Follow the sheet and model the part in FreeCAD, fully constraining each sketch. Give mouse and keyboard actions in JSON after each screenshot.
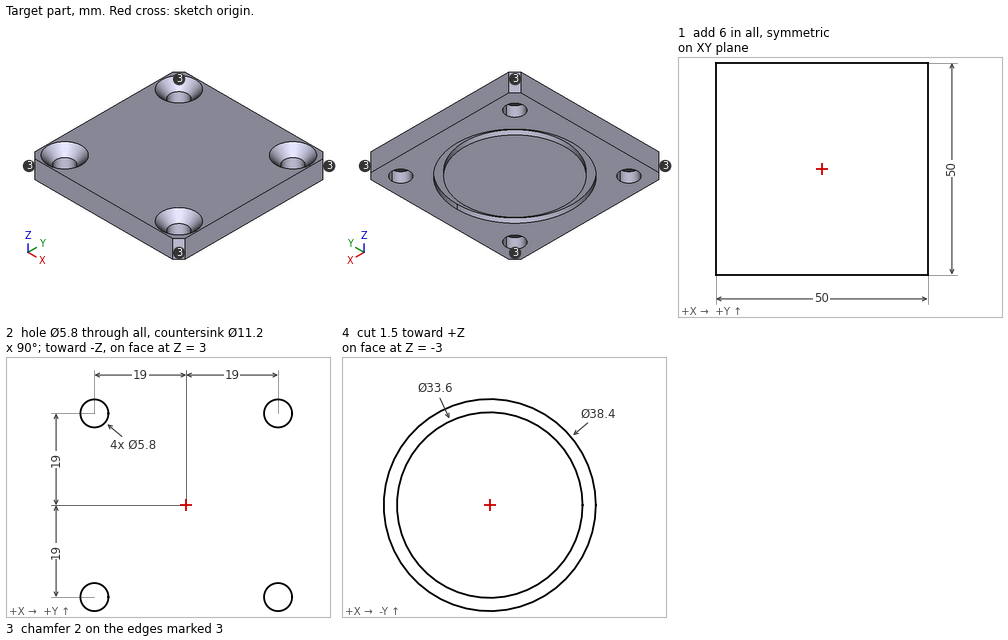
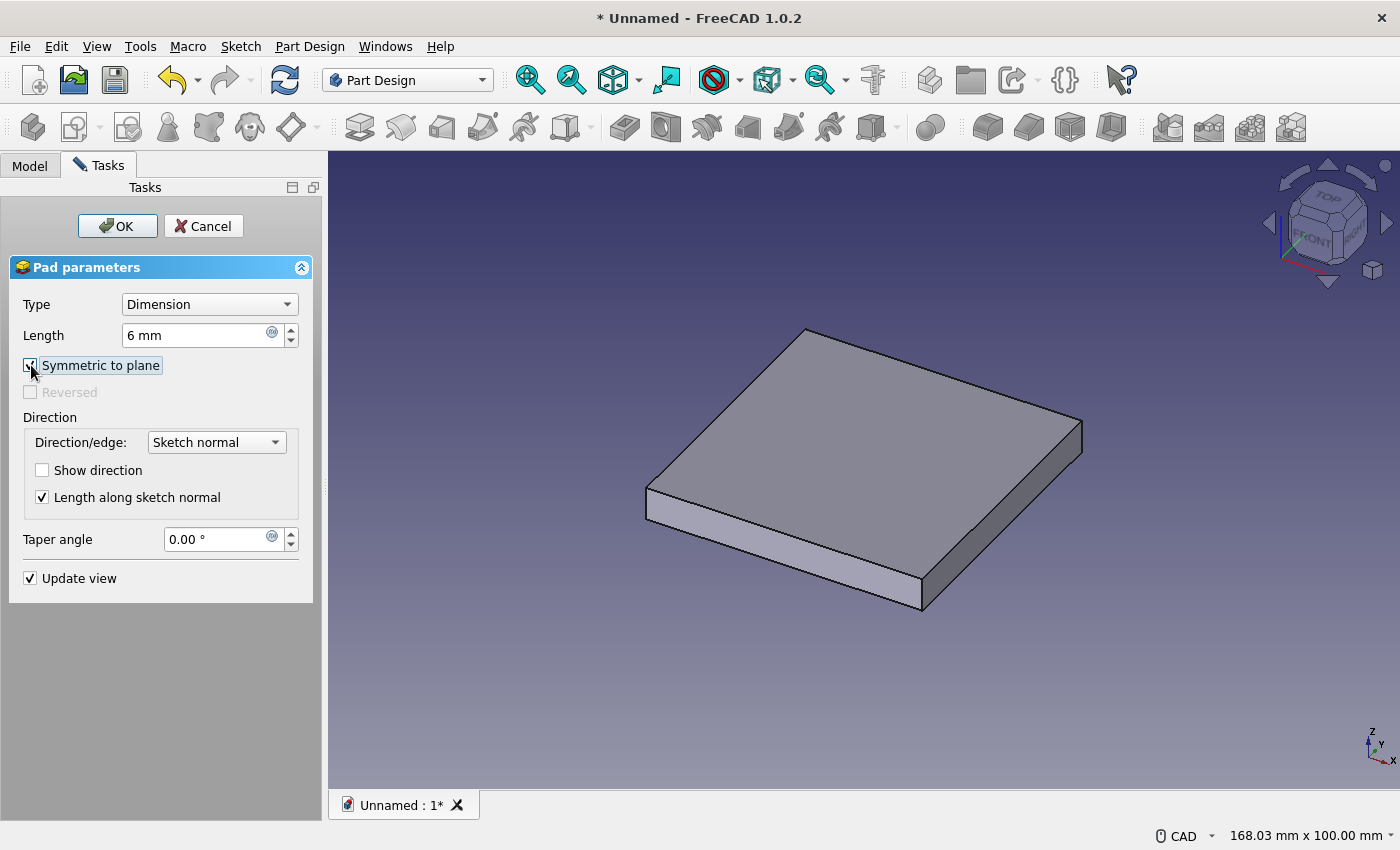
{"action": "left_click", "coordinate": [118, 226]}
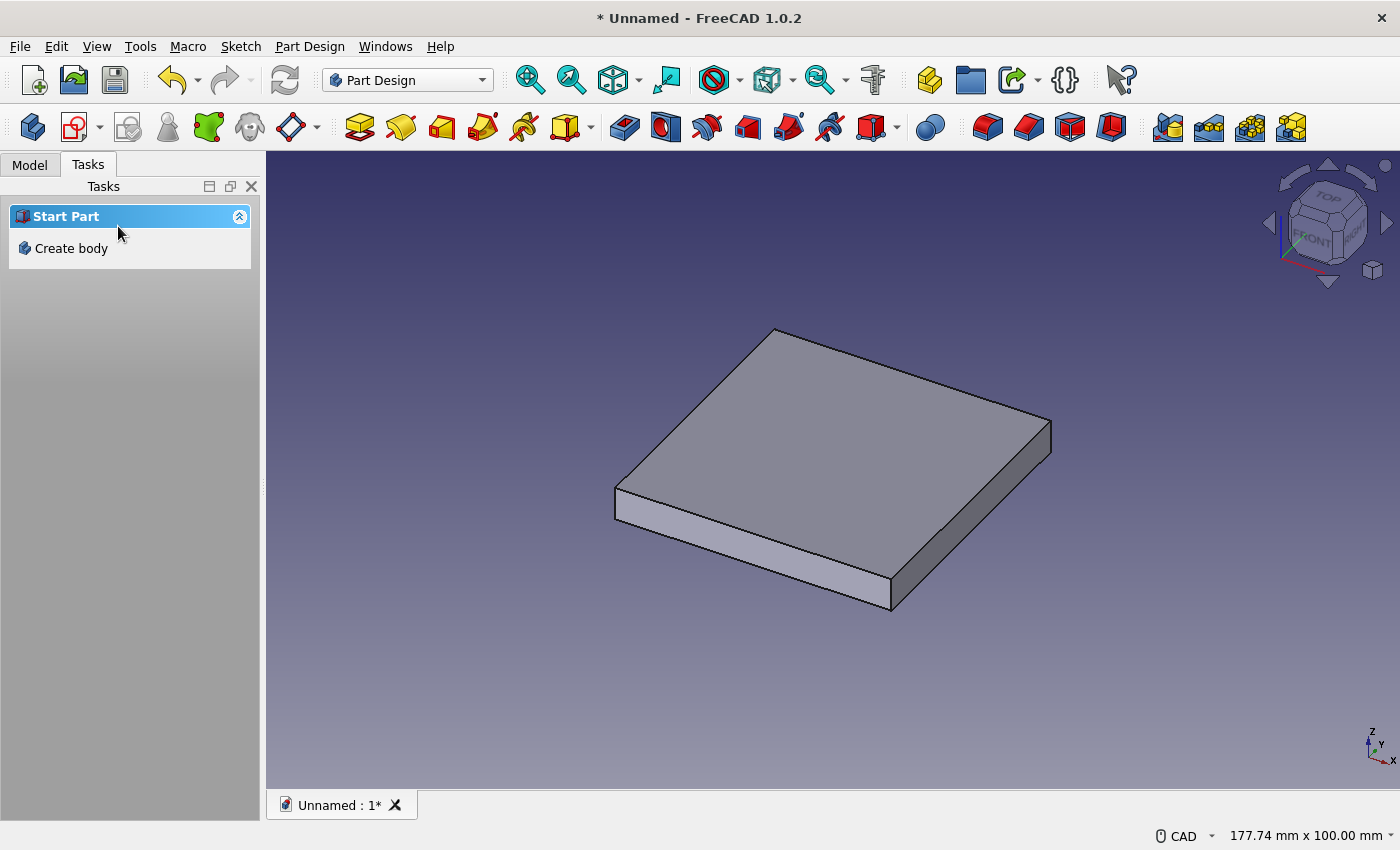
{"action": "left_click", "coordinate": [531, 80]}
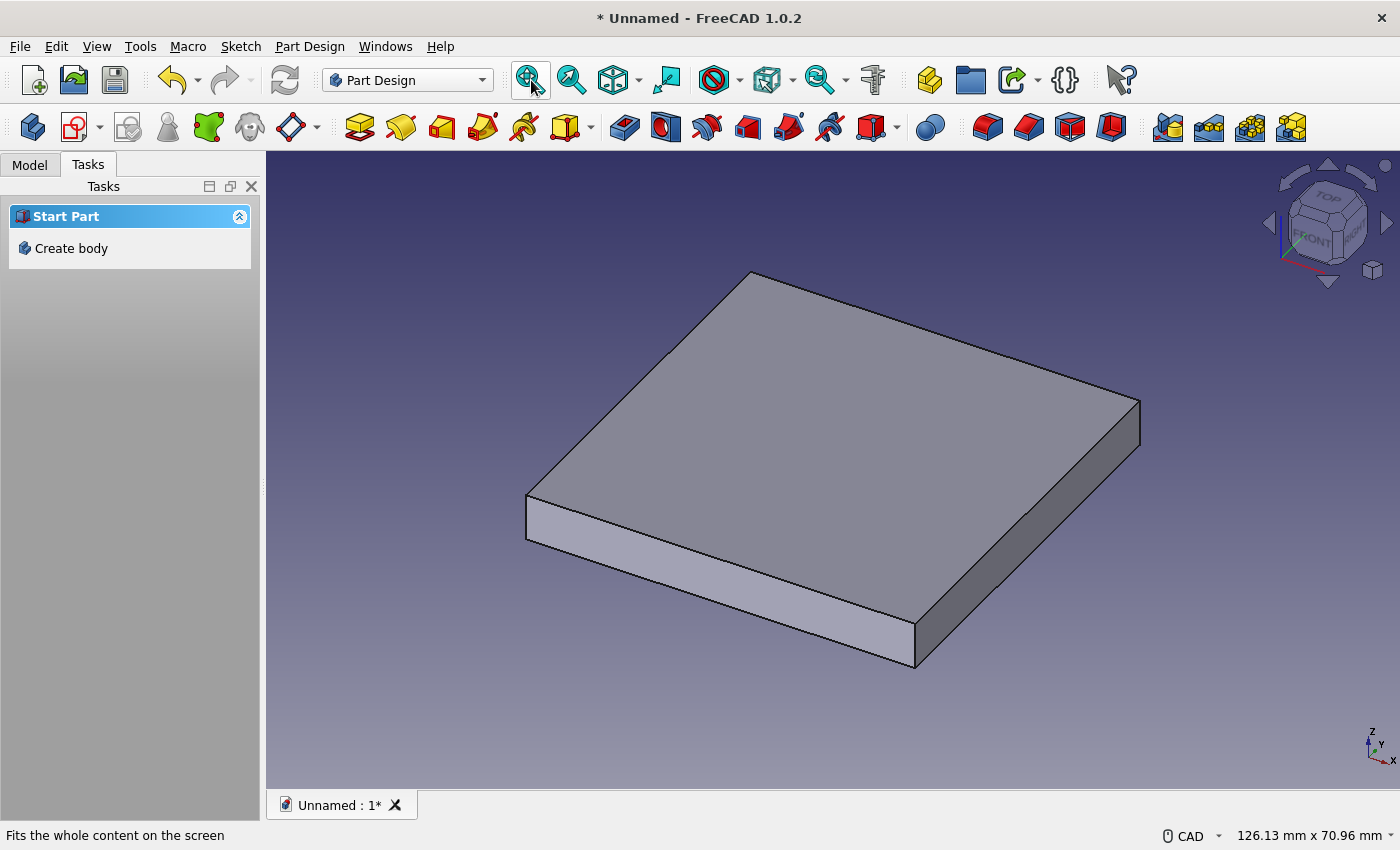
{"action": "left_click", "coordinate": [833, 447]}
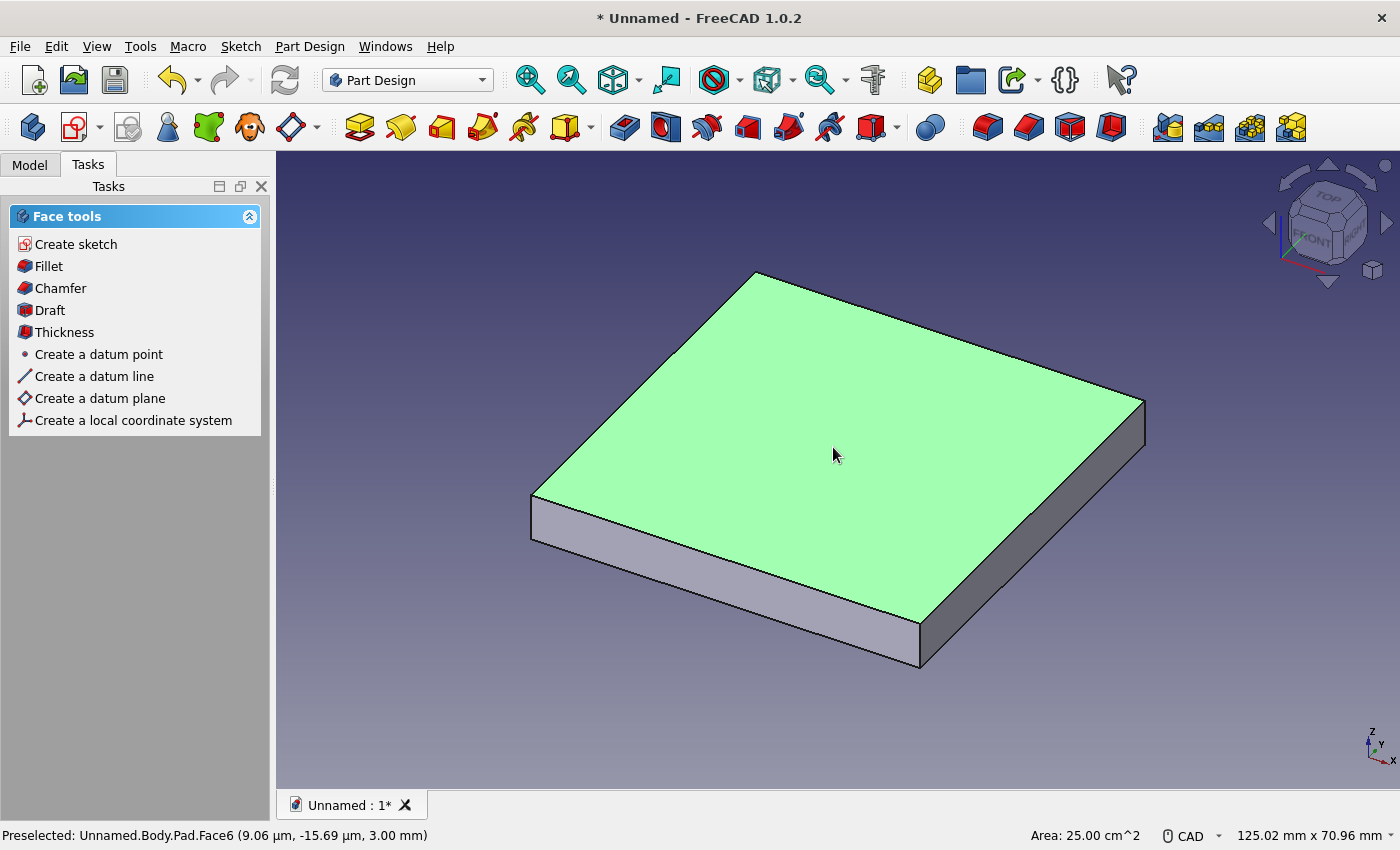
{"action": "left_click", "coordinate": [74, 128]}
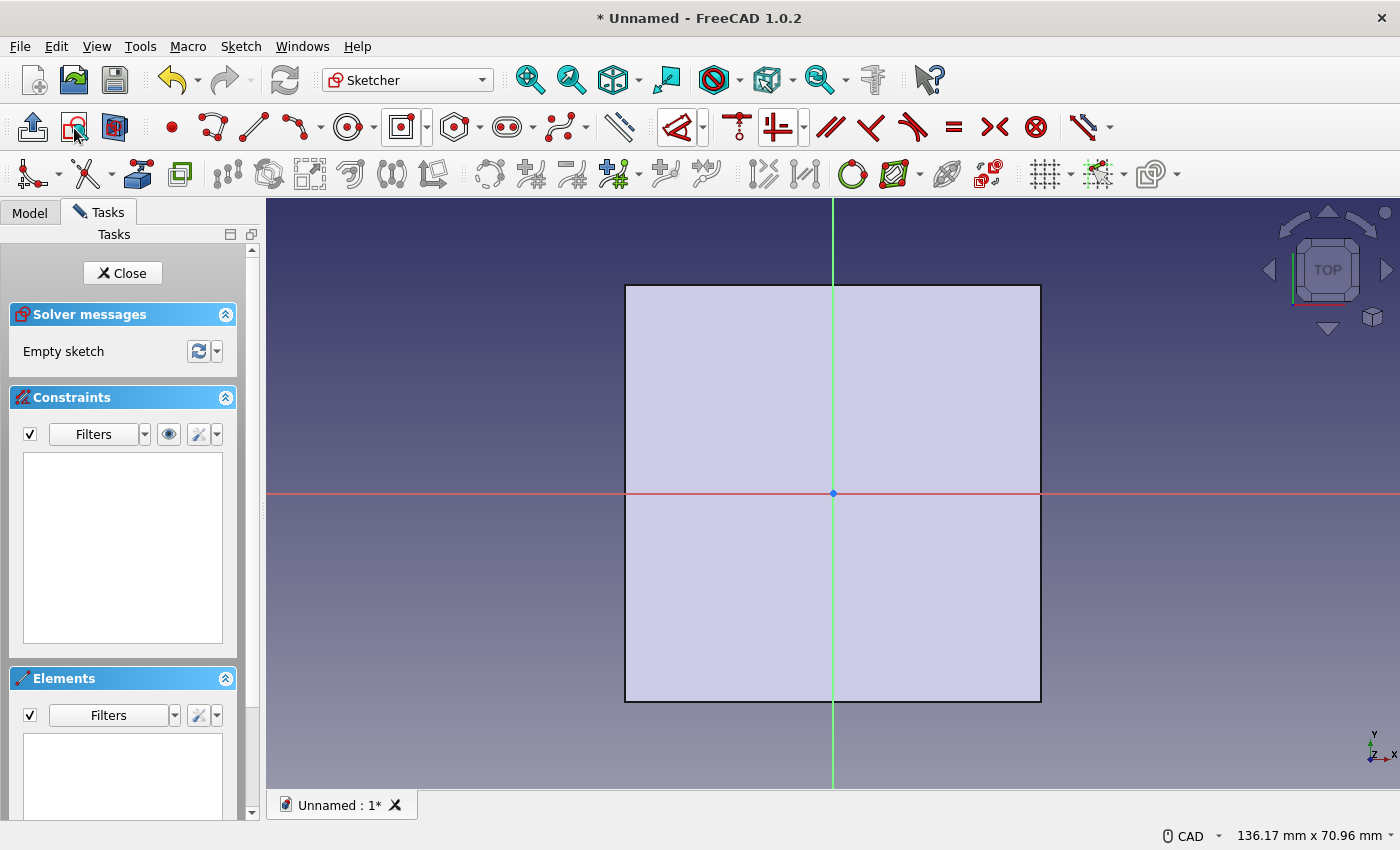
{"action": "left_click", "coordinate": [348, 128]}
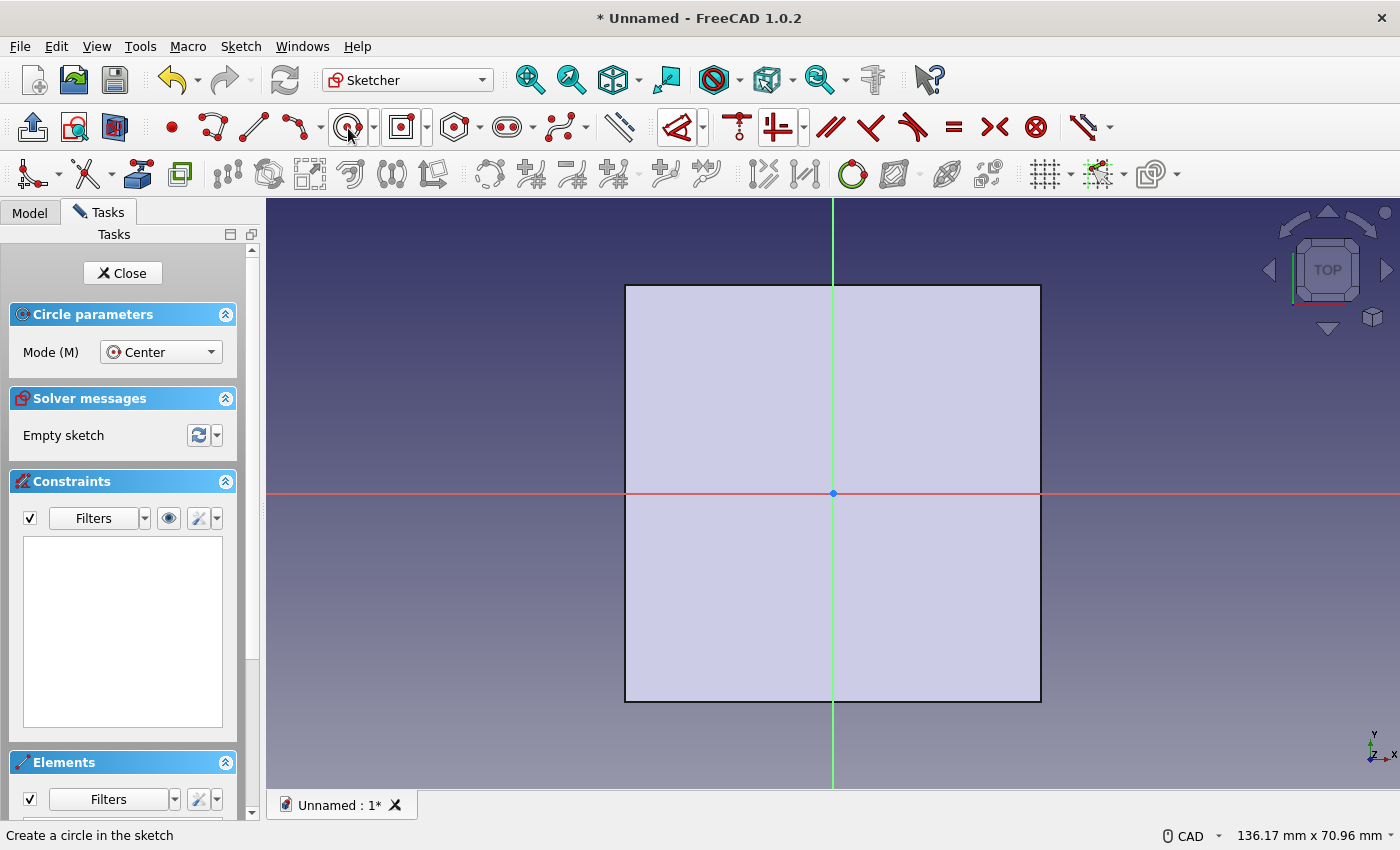
{"action": "left_click", "coordinate": [675, 335]}
{"action": "left_click", "coordinate": [692, 318]}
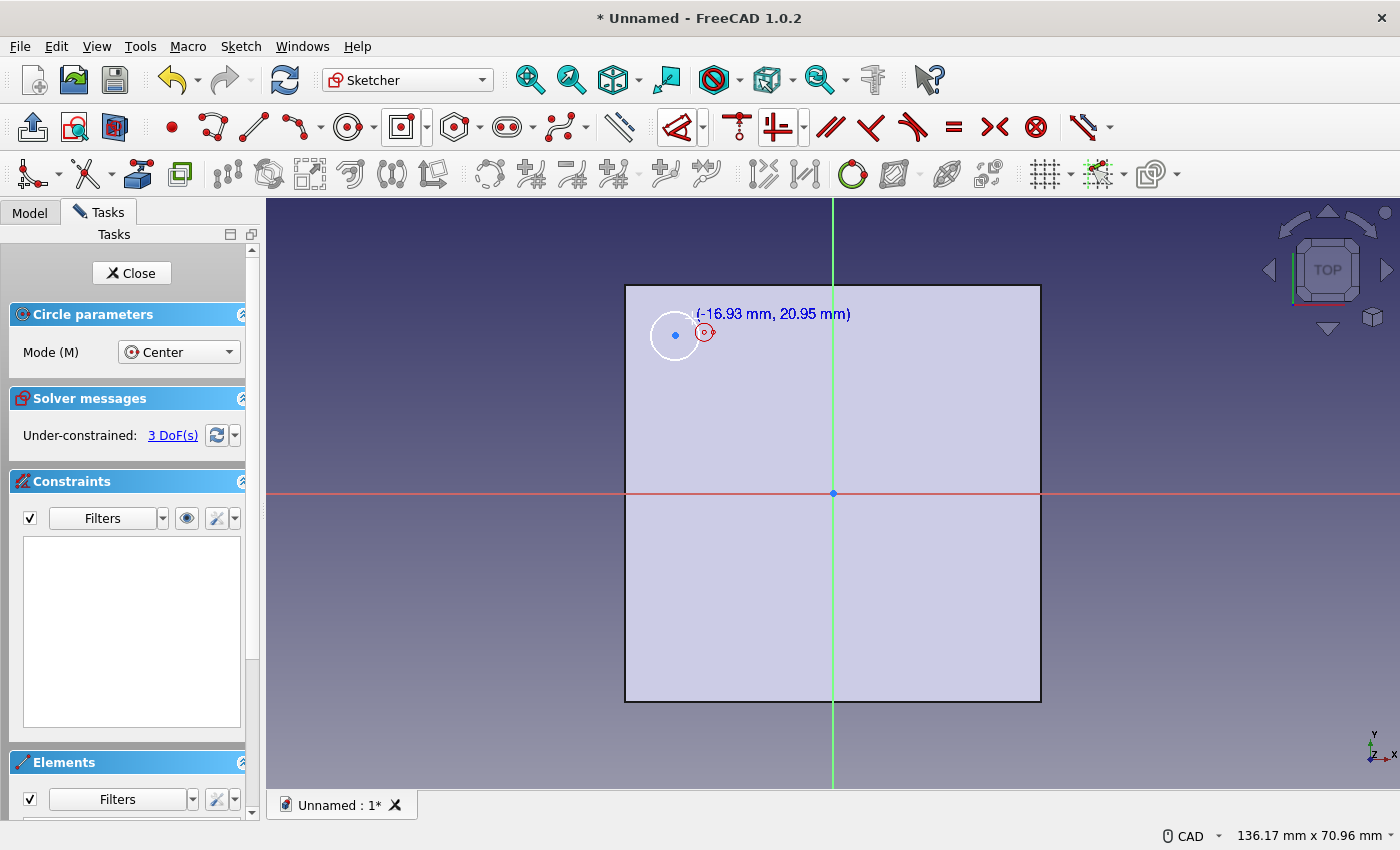
{"action": "left_click", "coordinate": [991, 335]}
{"action": "left_click", "coordinate": [1008, 318]}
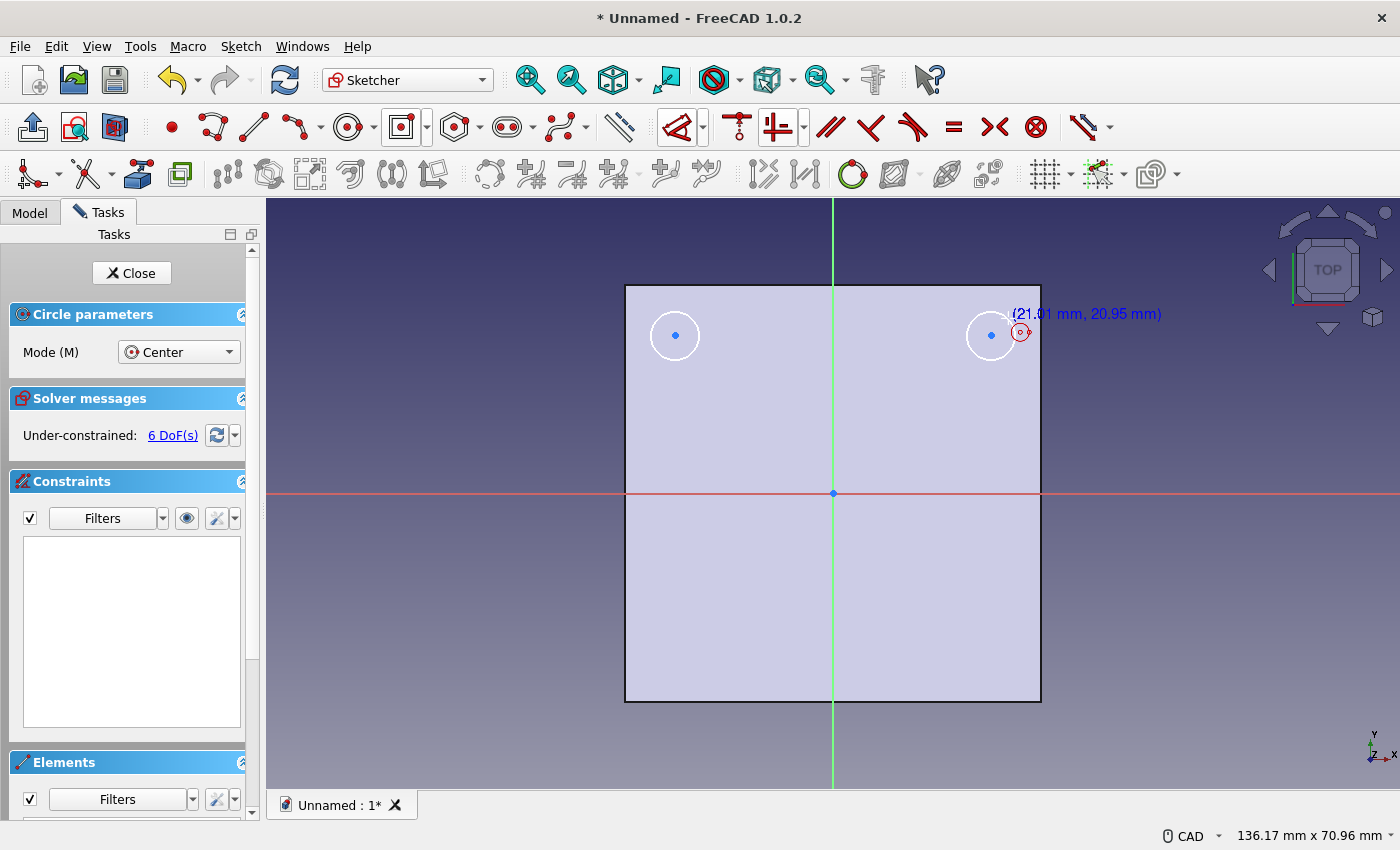
{"action": "left_click", "coordinate": [675, 652]}
{"action": "left_click", "coordinate": [692, 635]}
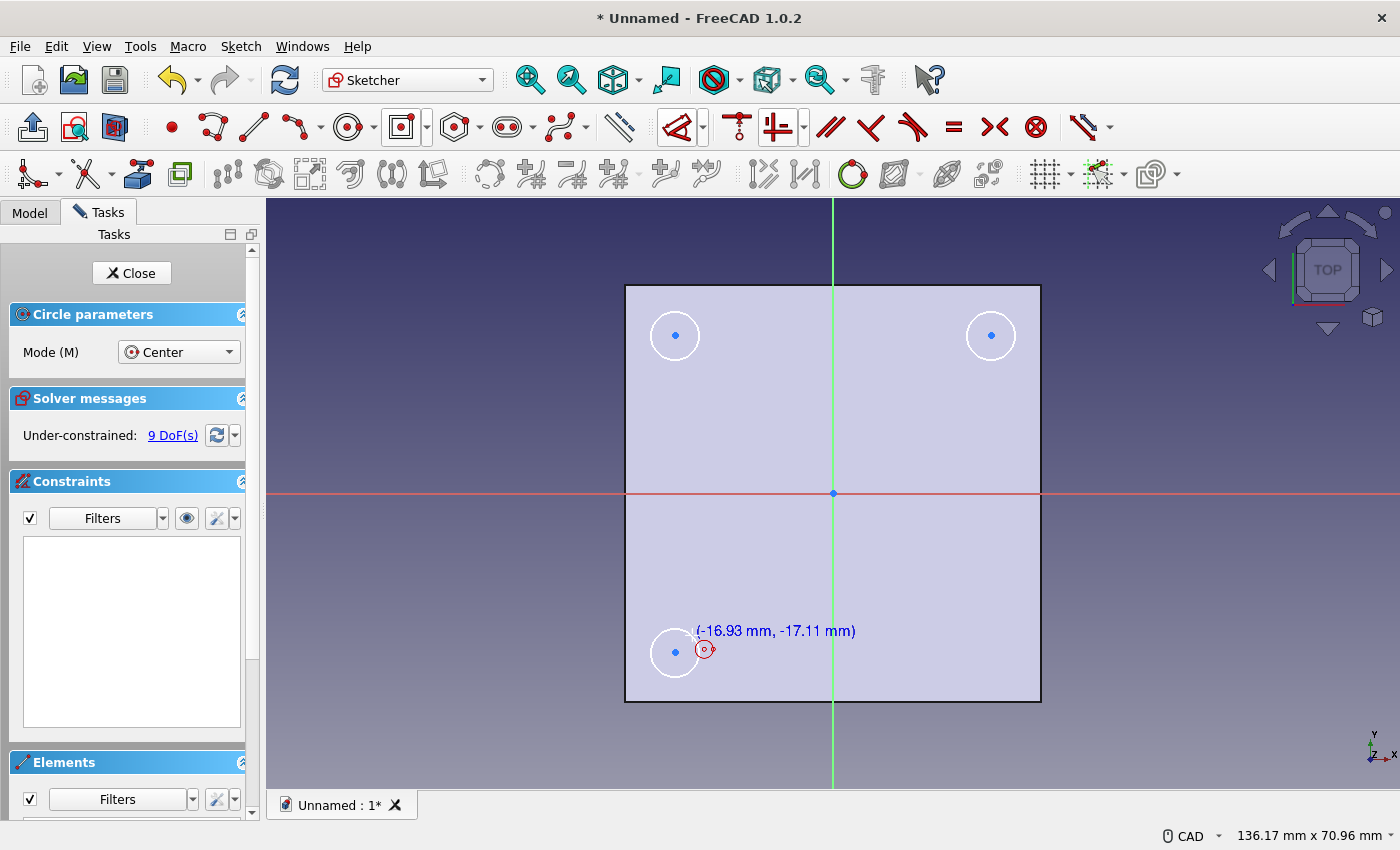
{"action": "left_click", "coordinate": [991, 652]}
{"action": "left_click", "coordinate": [1008, 635]}
{"action": "key", "text": "Escape"}